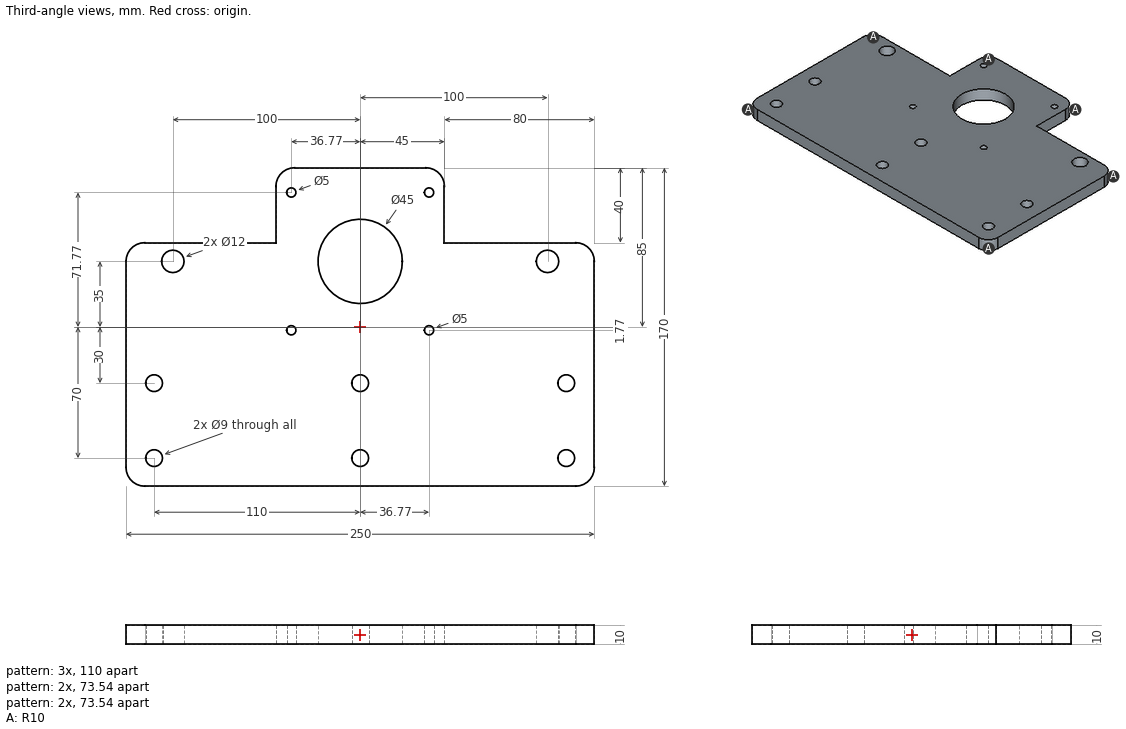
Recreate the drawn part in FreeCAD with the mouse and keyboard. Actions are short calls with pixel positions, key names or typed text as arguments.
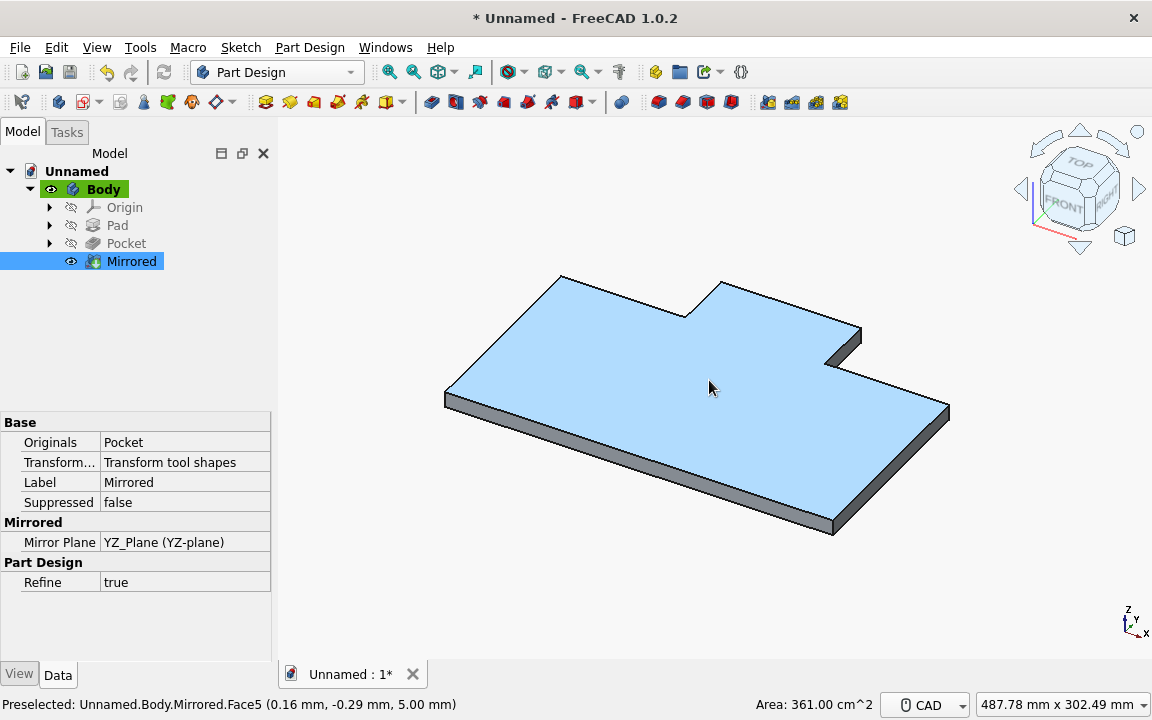
click(84, 102)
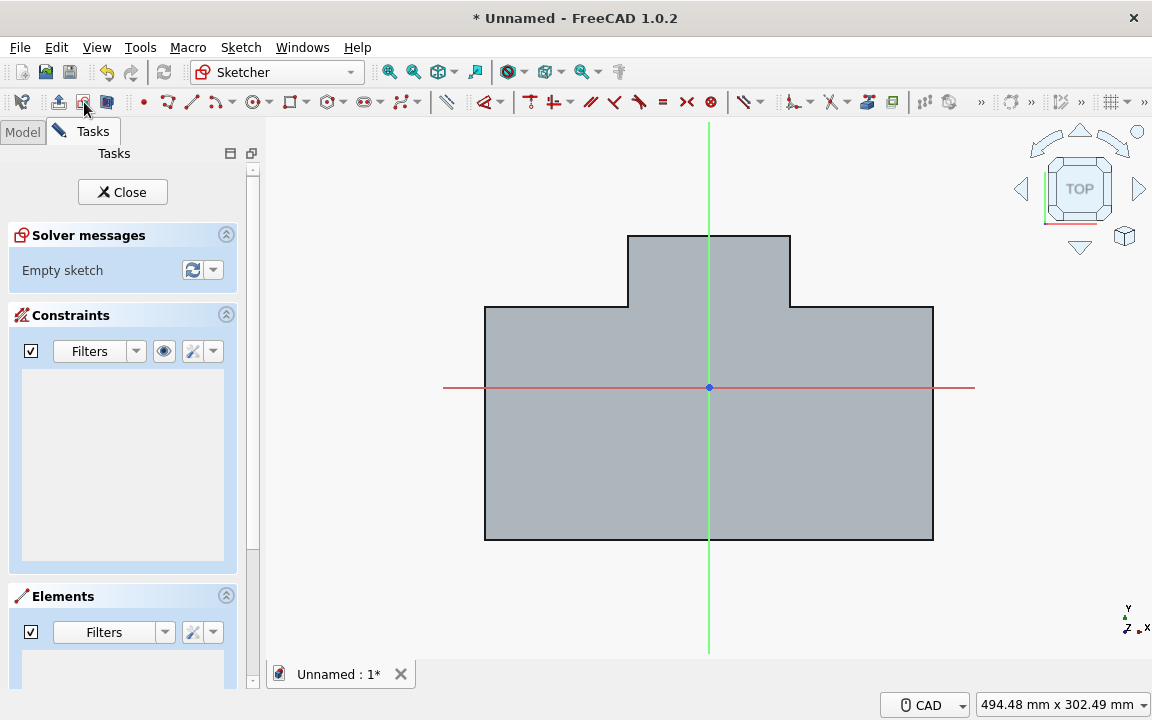
scroll(579, 509, up, 4)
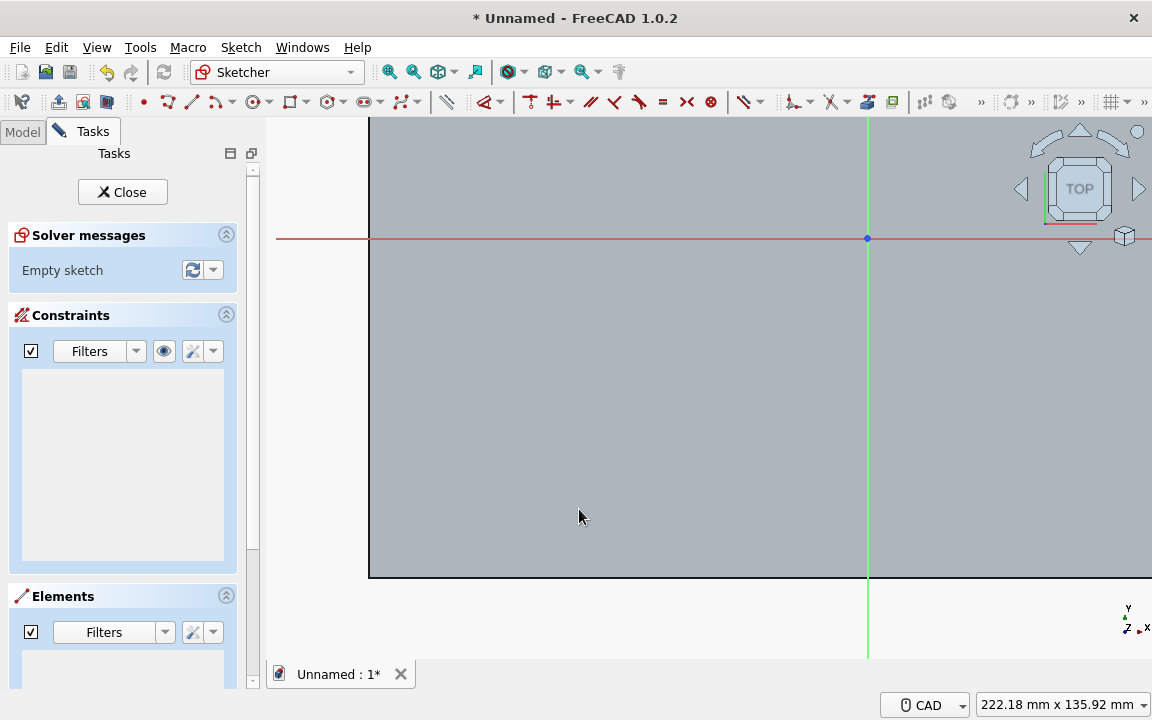
key(g)
key(c)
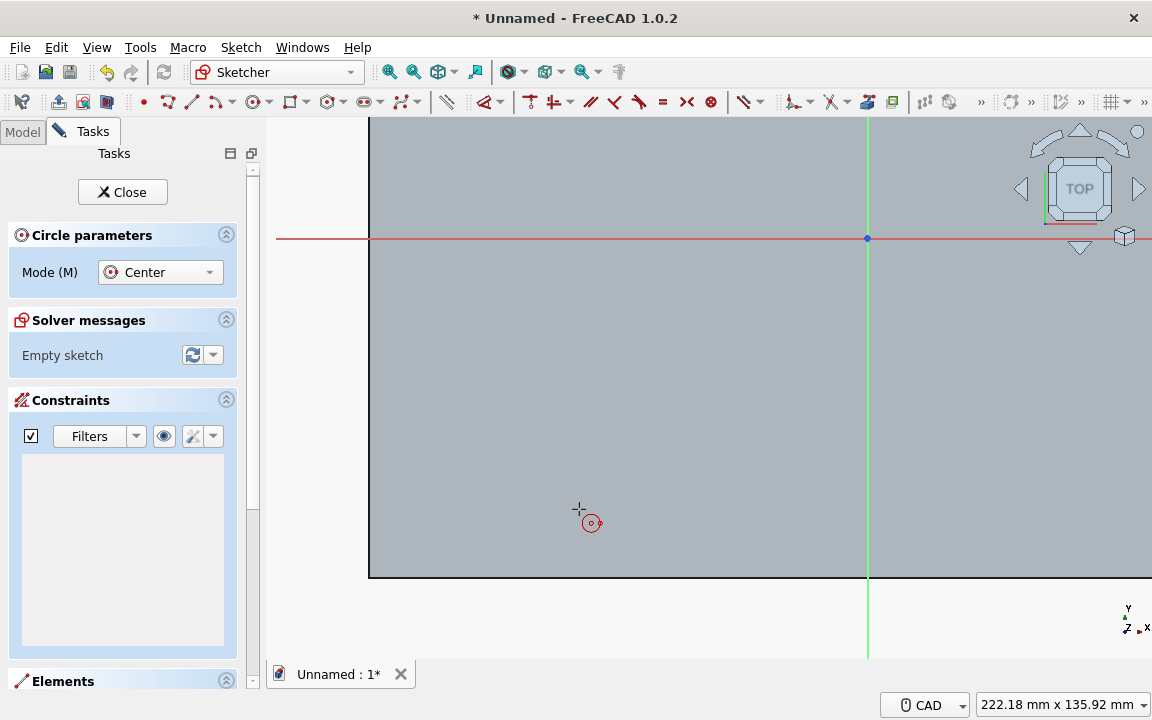
scroll(429, 518, up, 2)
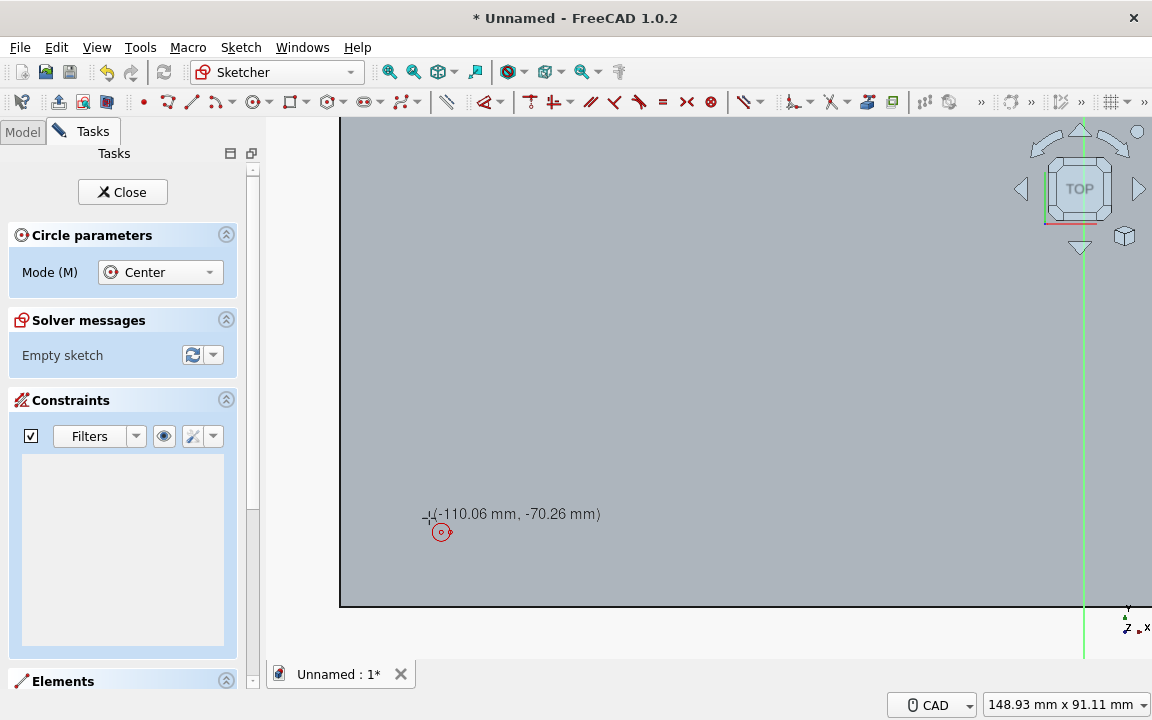
click(429, 518)
move(448, 499)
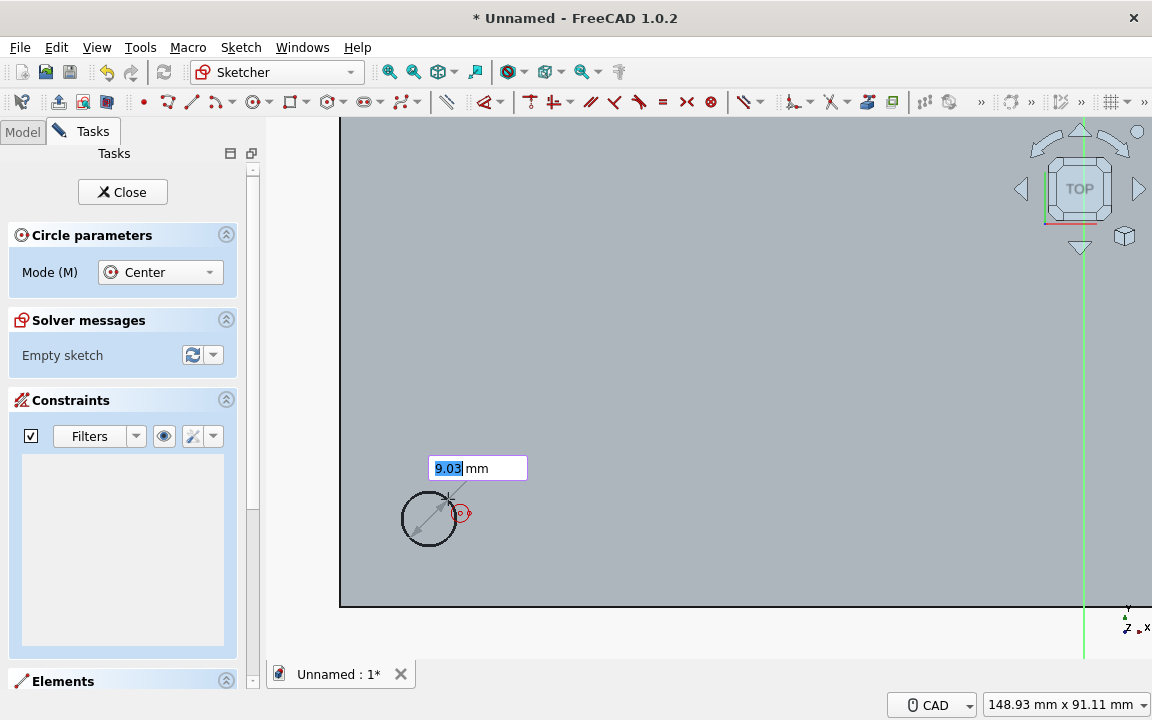
text(9)
key(Return)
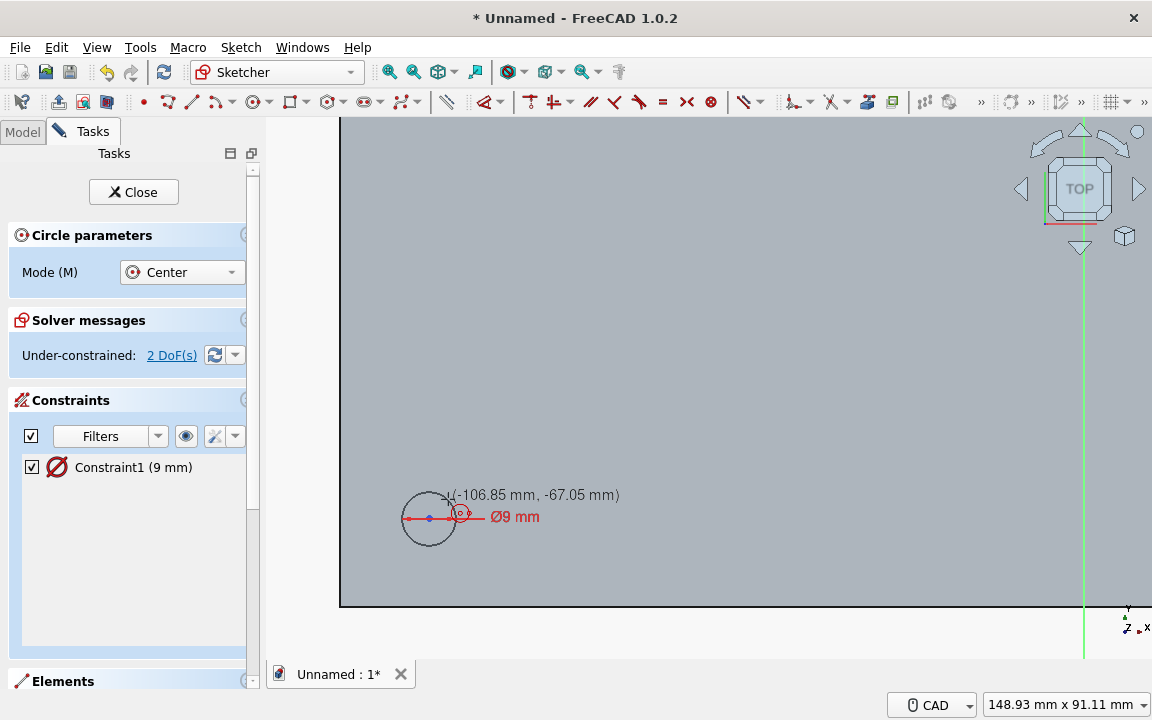
click(429, 280)
move(448, 261)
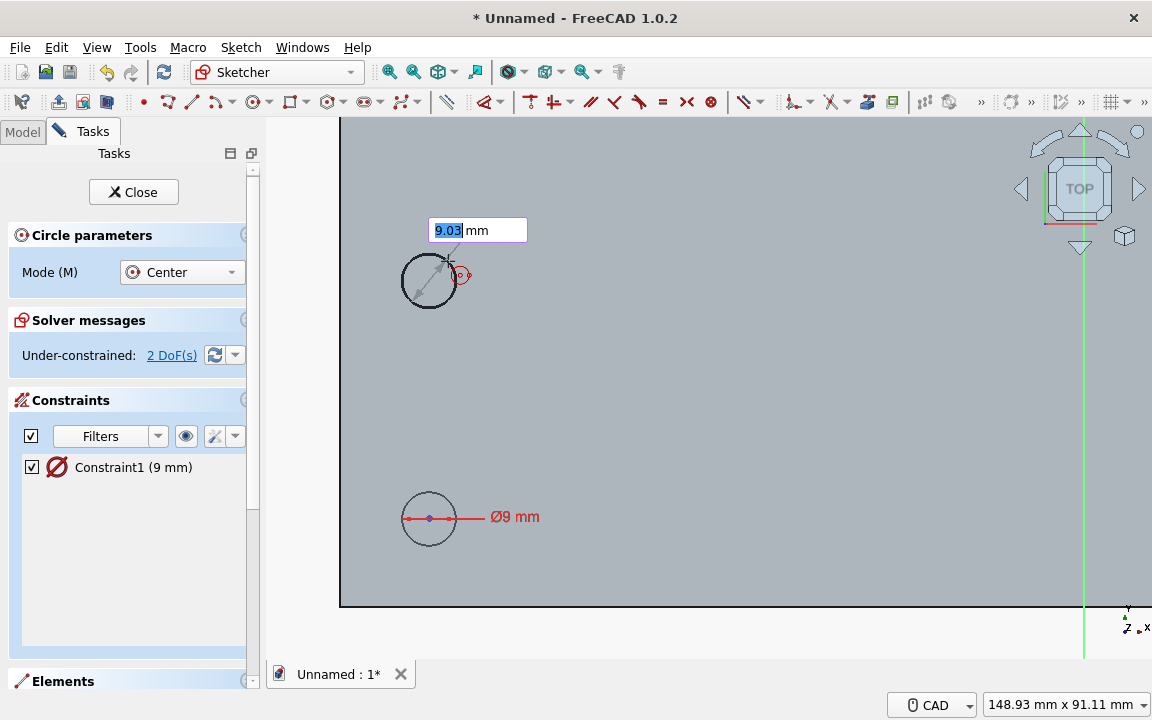
text(9)
key(Return)
key(Escape)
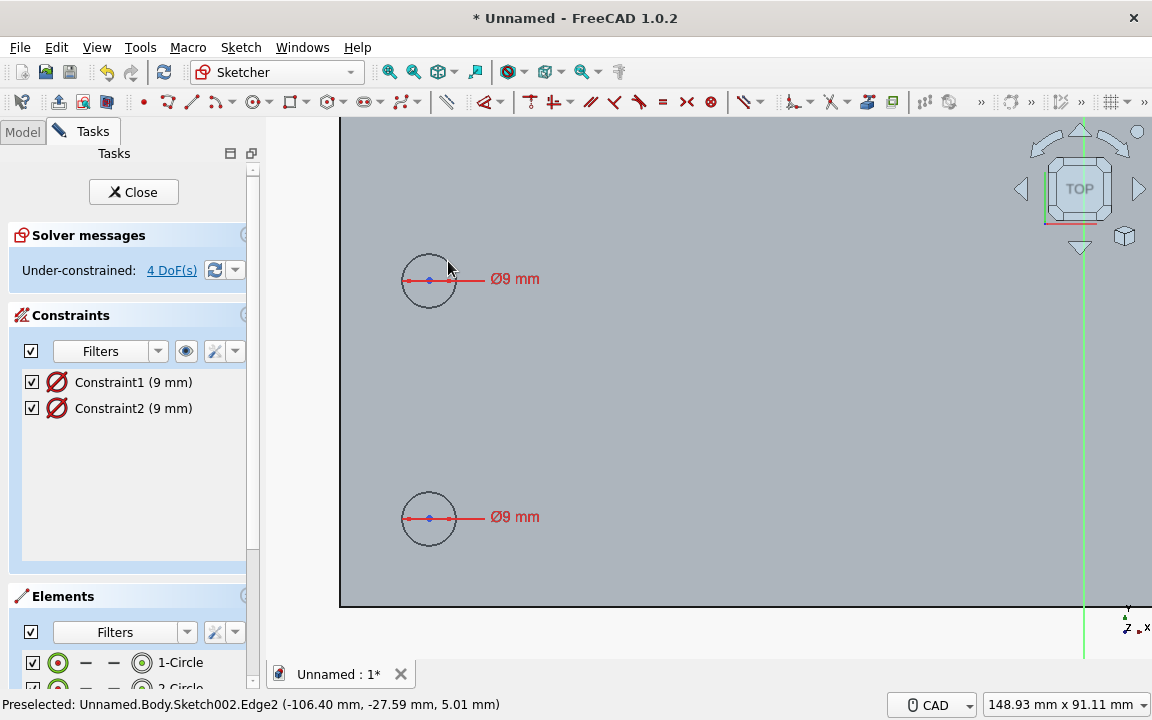
click(429, 519)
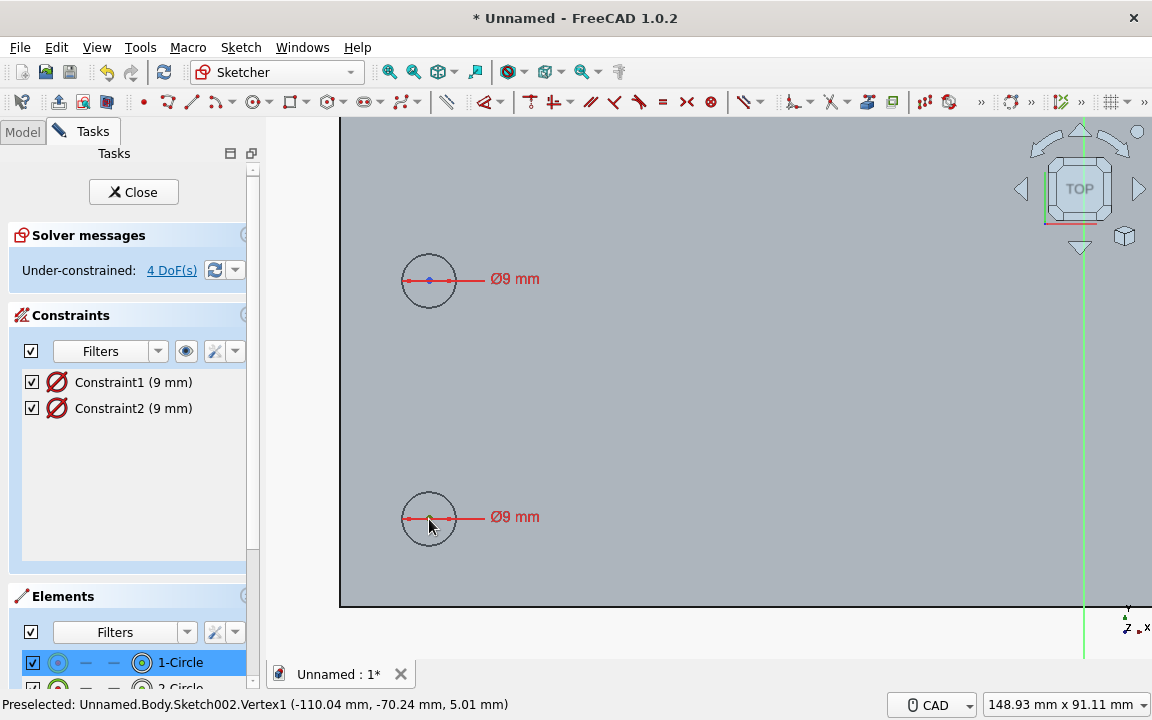
click(429, 281)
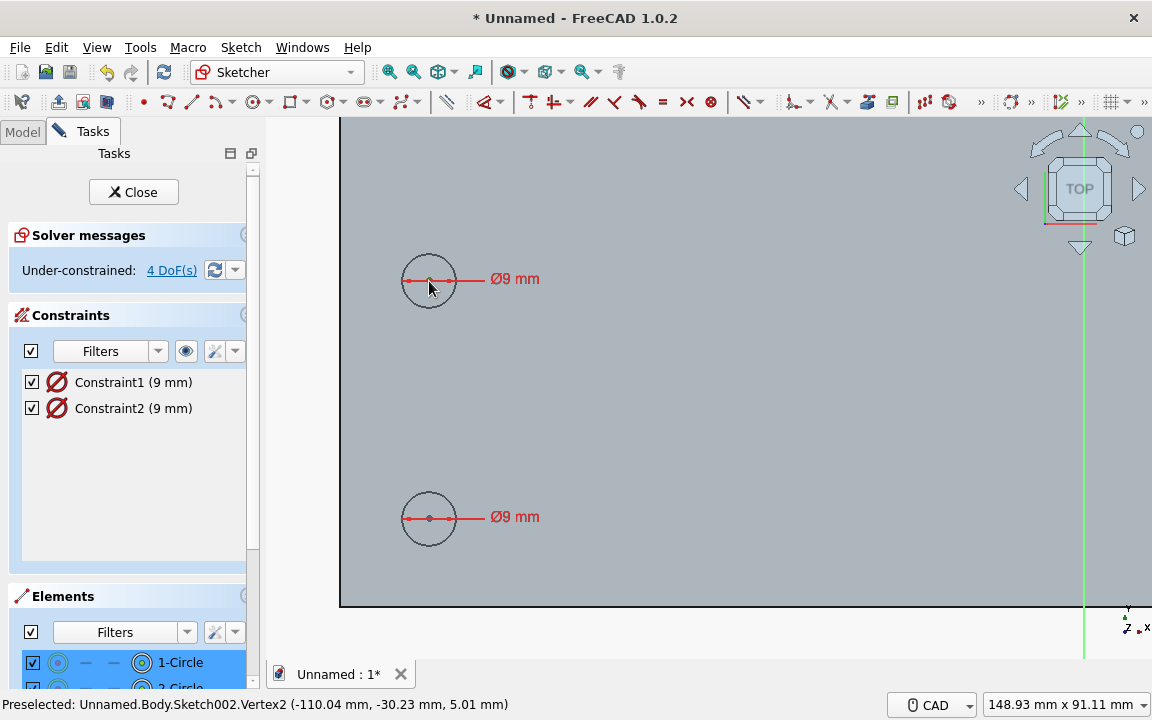
key(v)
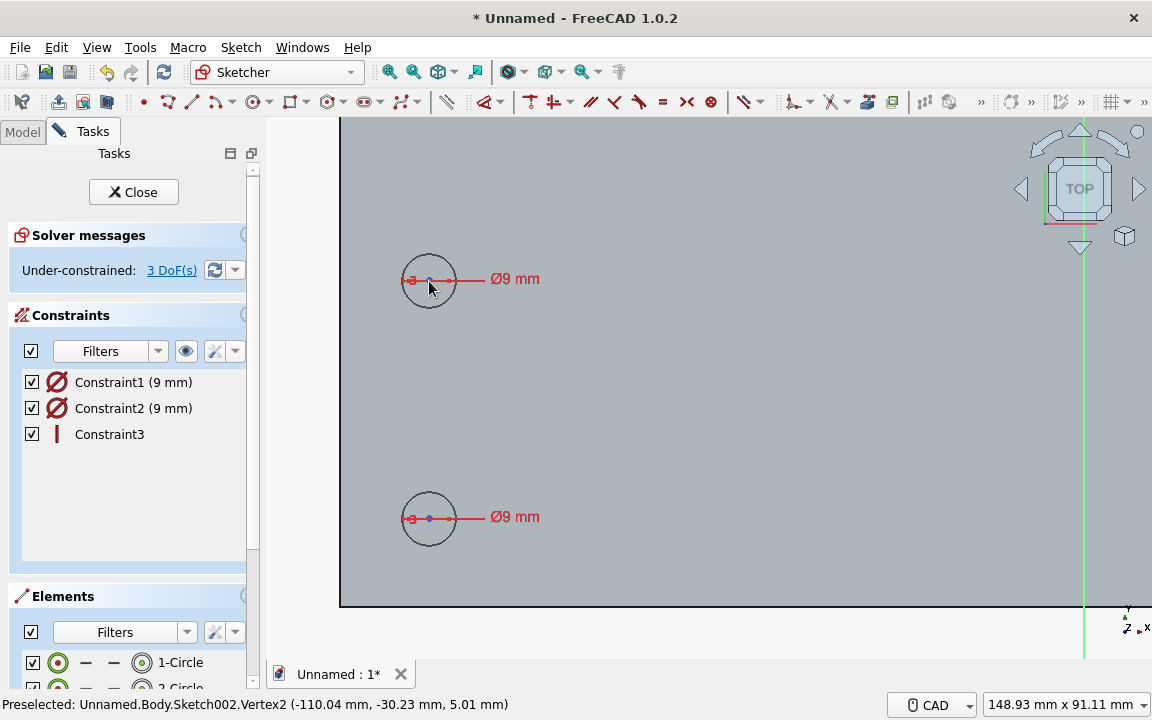
click(484, 102)